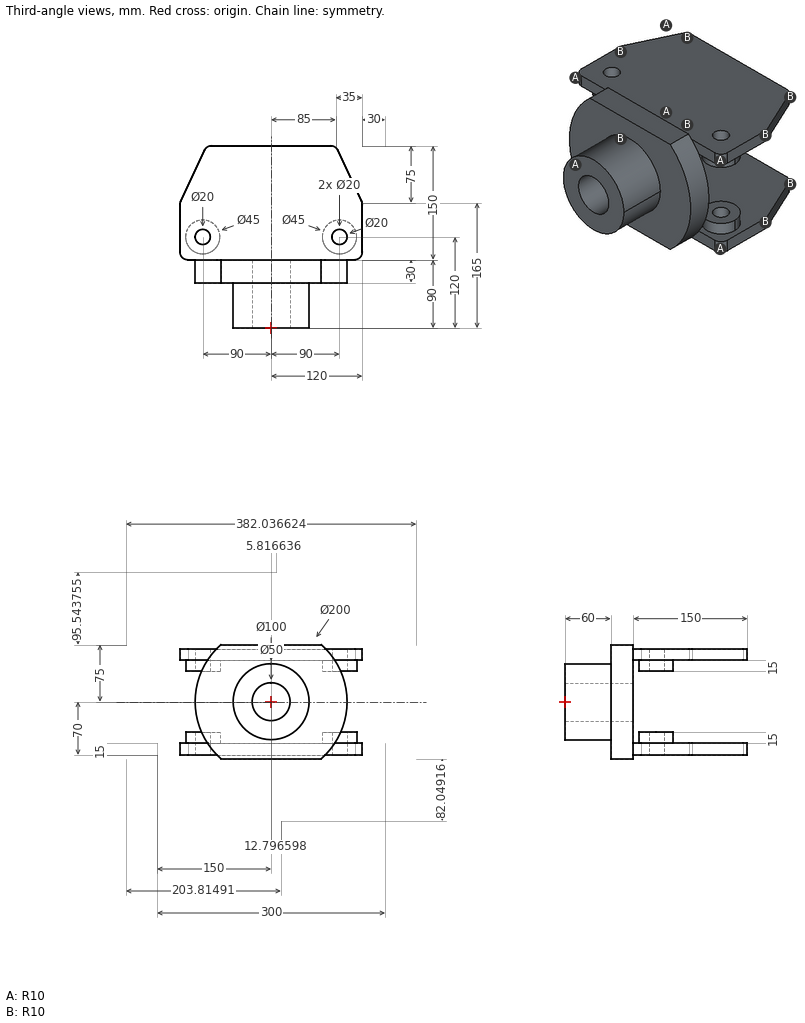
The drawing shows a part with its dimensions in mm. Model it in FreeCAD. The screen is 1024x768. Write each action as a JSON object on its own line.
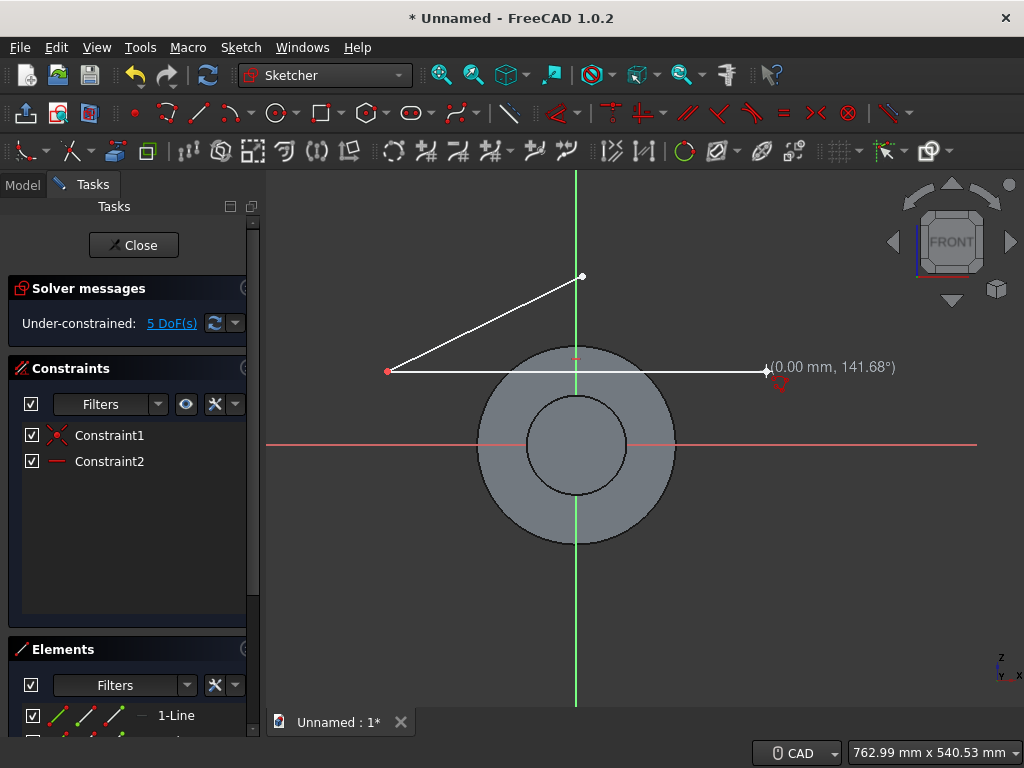
{"action": "scroll", "coordinate": [582, 276], "scroll_direction": "up", "scroll_amount": 6}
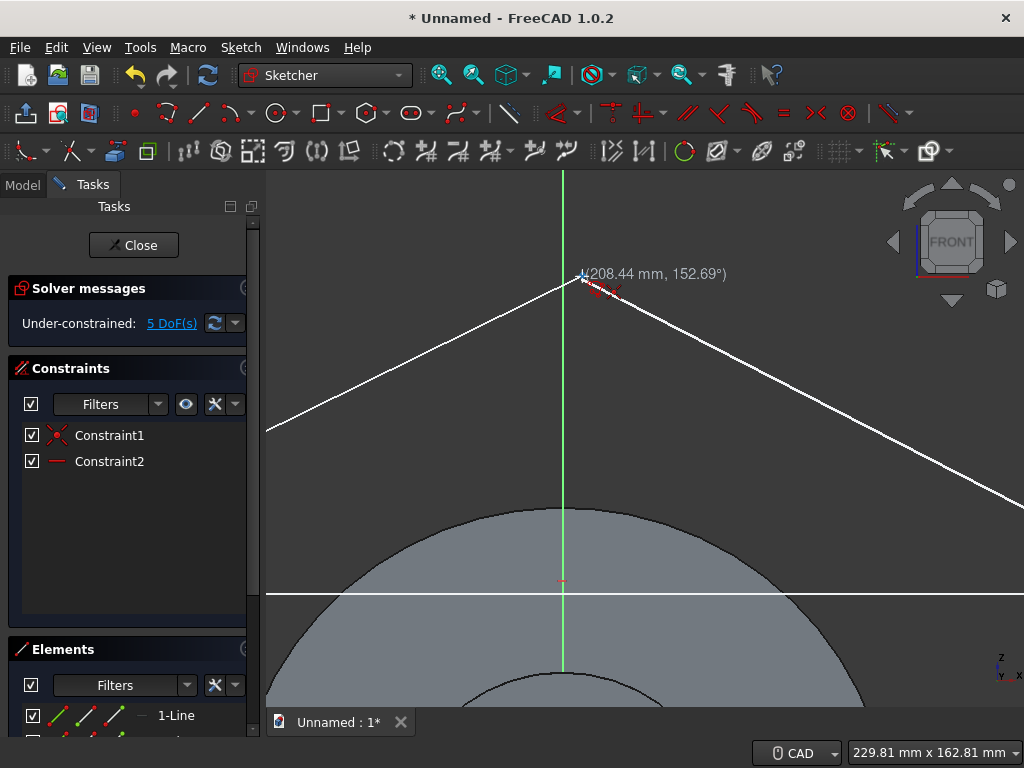
{"action": "left_click", "coordinate": [582, 276]}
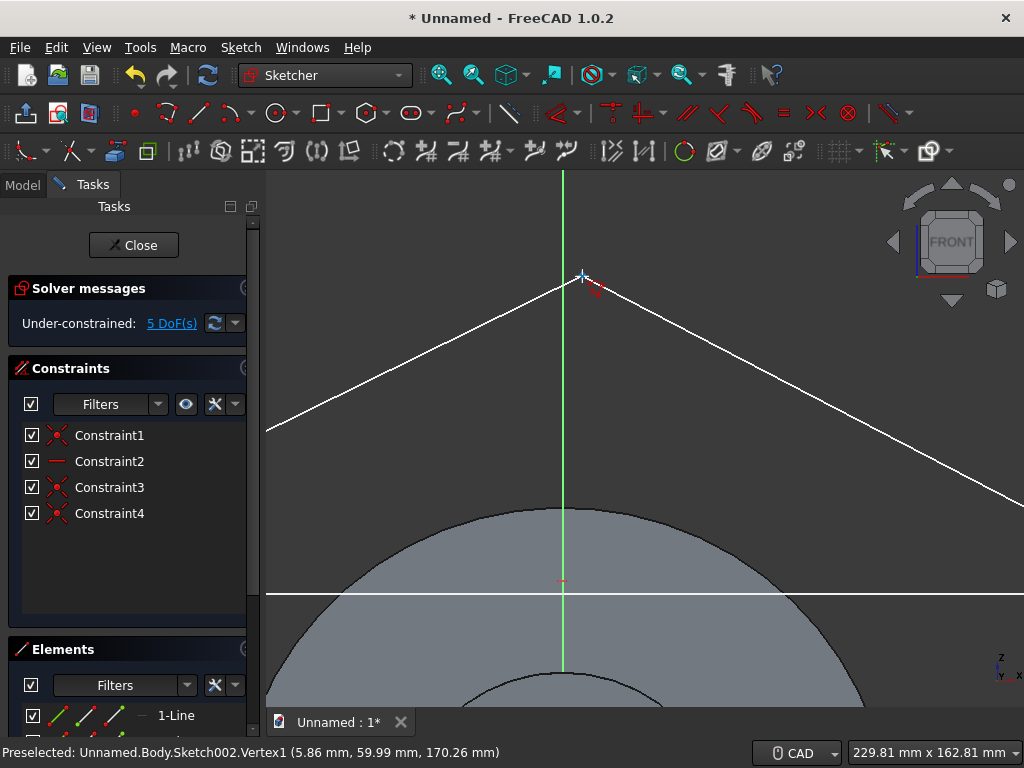
{"action": "scroll", "coordinate": [582, 276], "scroll_direction": "down", "scroll_amount": 6}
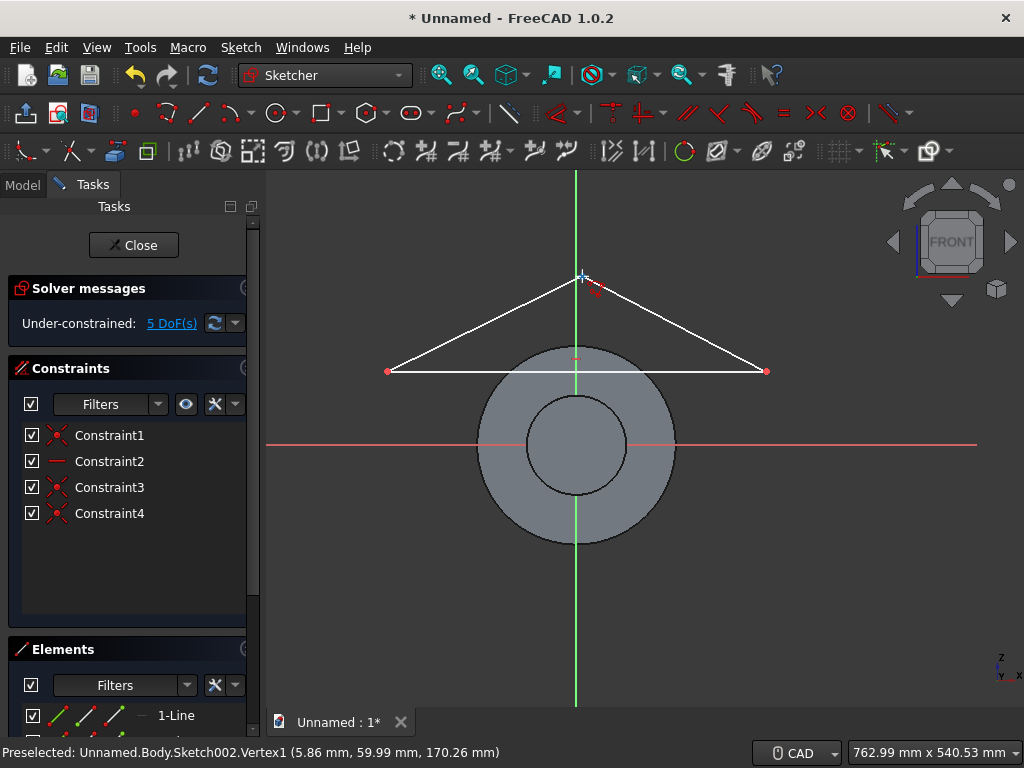
{"action": "scroll", "coordinate": [589, 601], "scroll_direction": "up", "scroll_amount": 2}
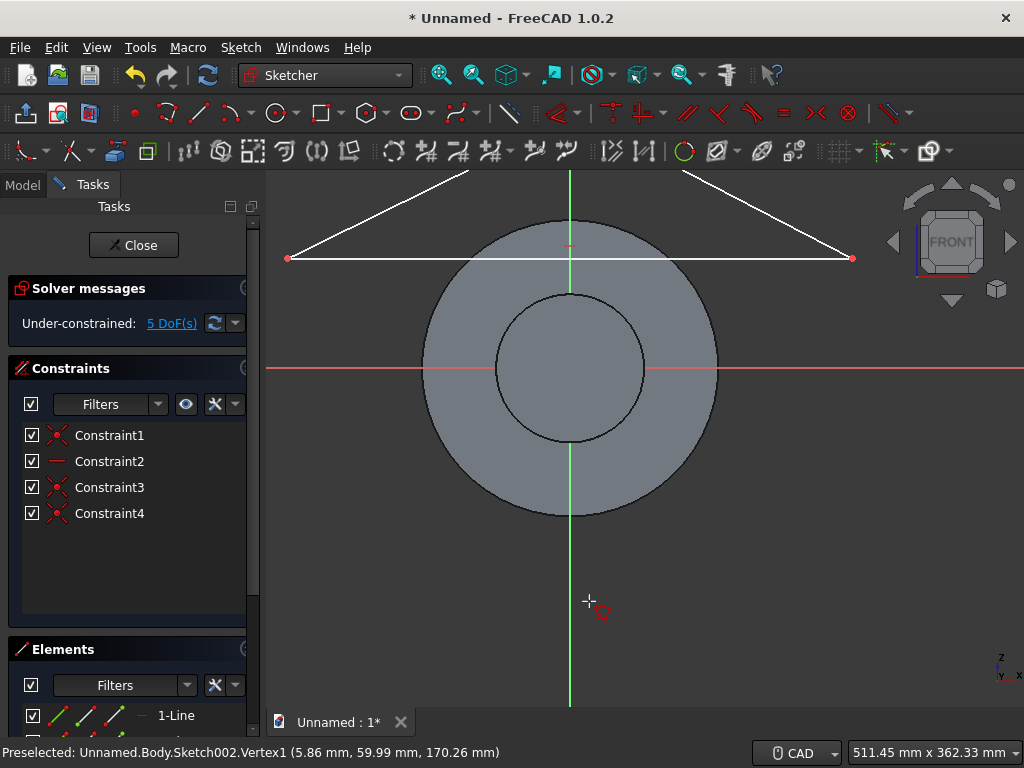
{"action": "left_click", "coordinate": [589, 601]}
{"action": "left_click", "coordinate": [853, 479]}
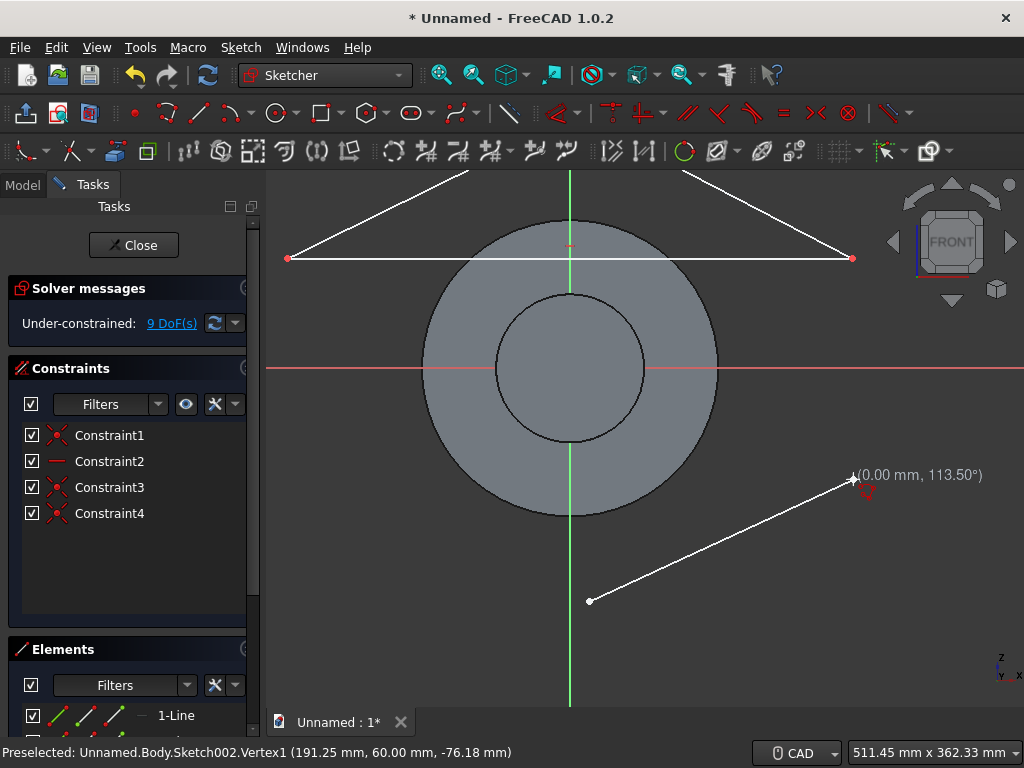
{"action": "scroll", "coordinate": [590, 602], "scroll_direction": "down", "scroll_amount": 2}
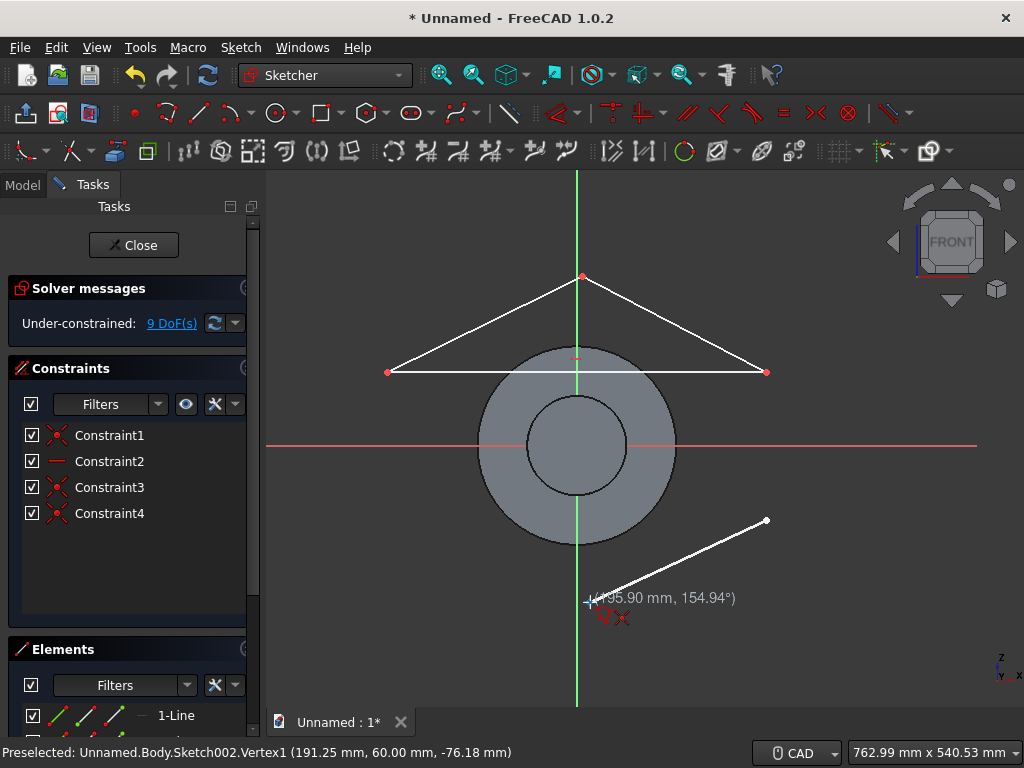
{"action": "left_click", "coordinate": [387, 520]}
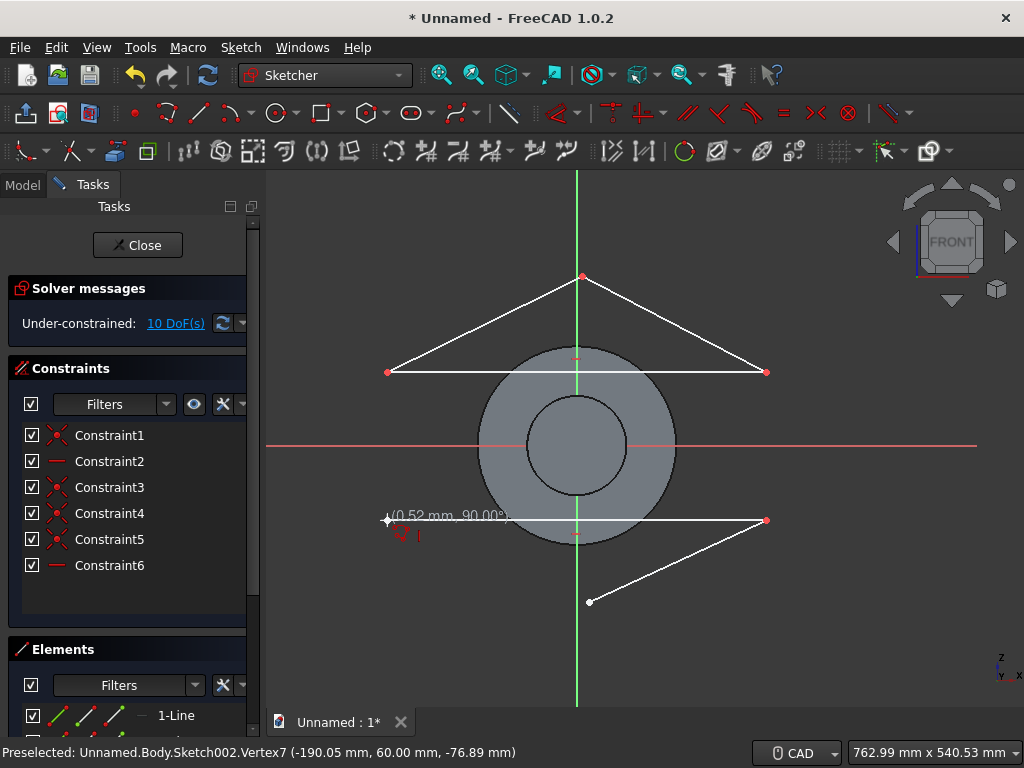
{"action": "scroll", "coordinate": [590, 602], "scroll_direction": "up", "scroll_amount": 2}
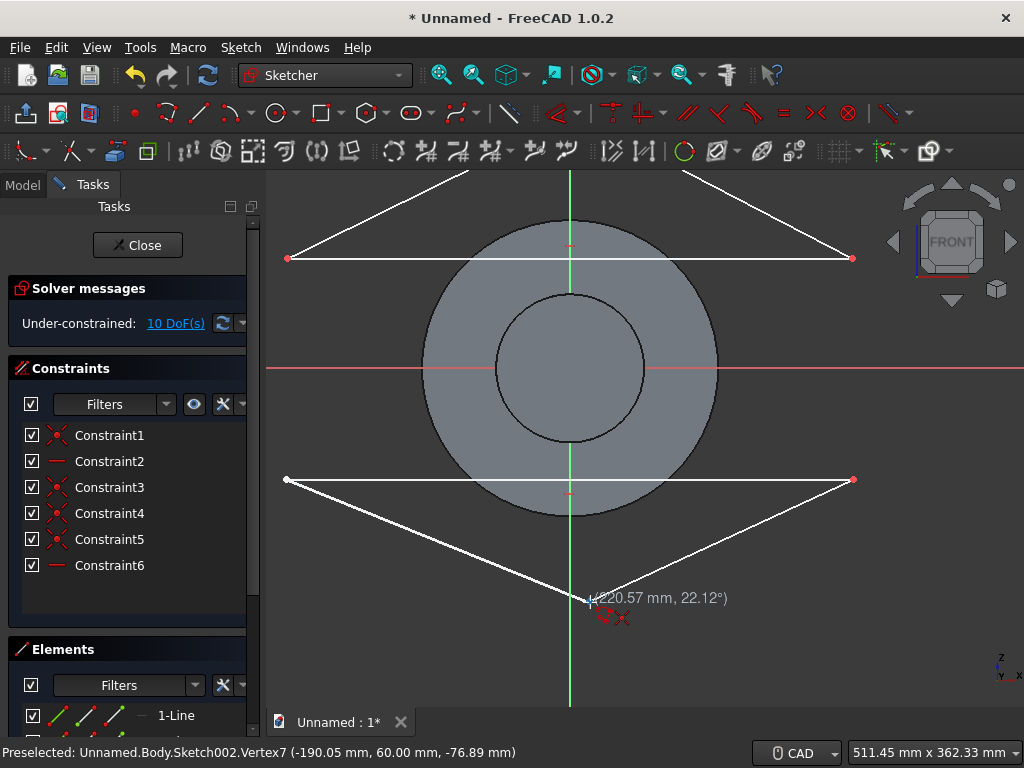
{"action": "left_click", "coordinate": [589, 602]}
{"action": "key", "text": "Escape"}
{"action": "key", "text": "Escape"}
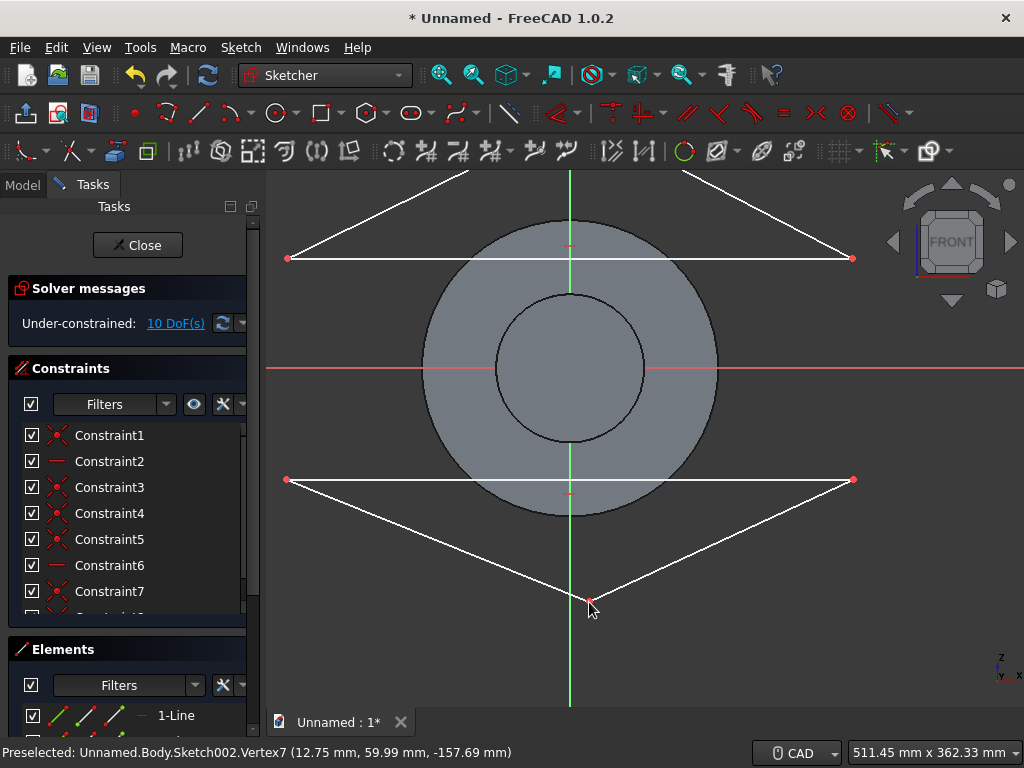
{"action": "left_click", "coordinate": [853, 259]}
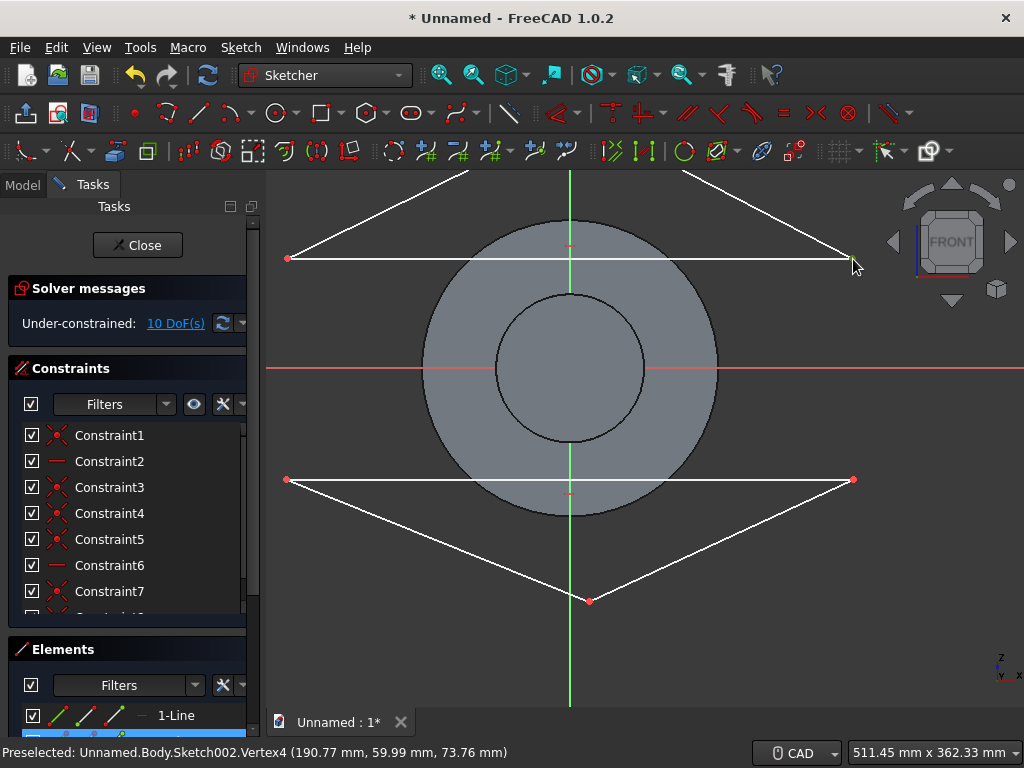
{"action": "left_click", "coordinate": [853, 480]}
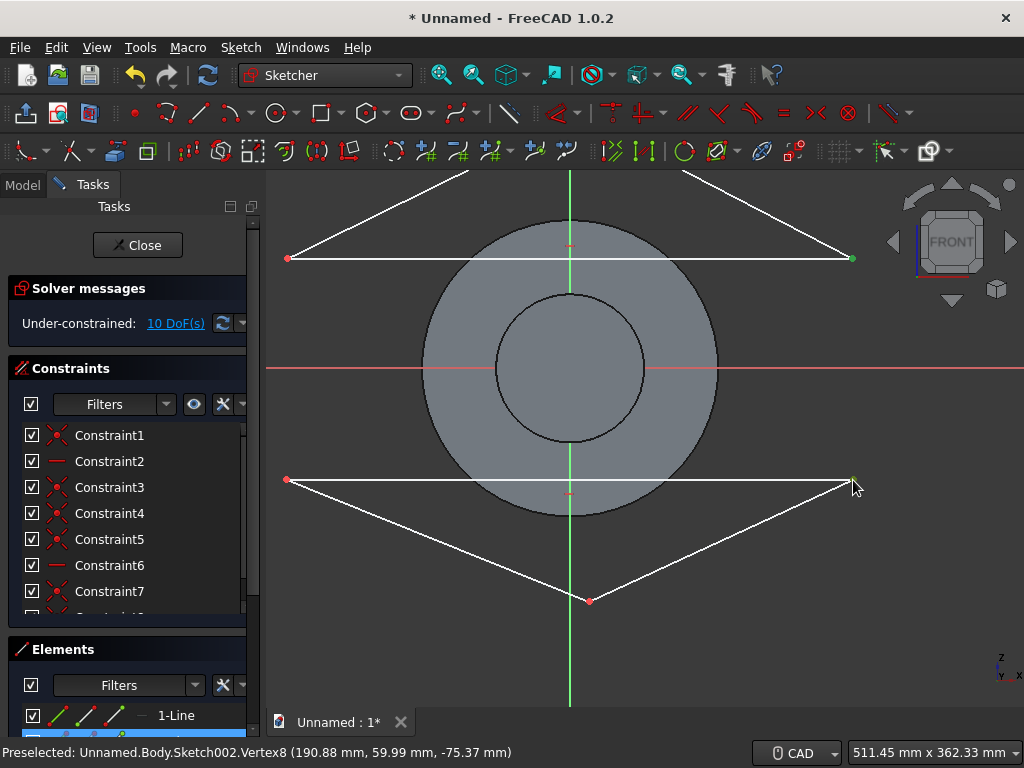
{"action": "left_click", "coordinate": [334, 368]}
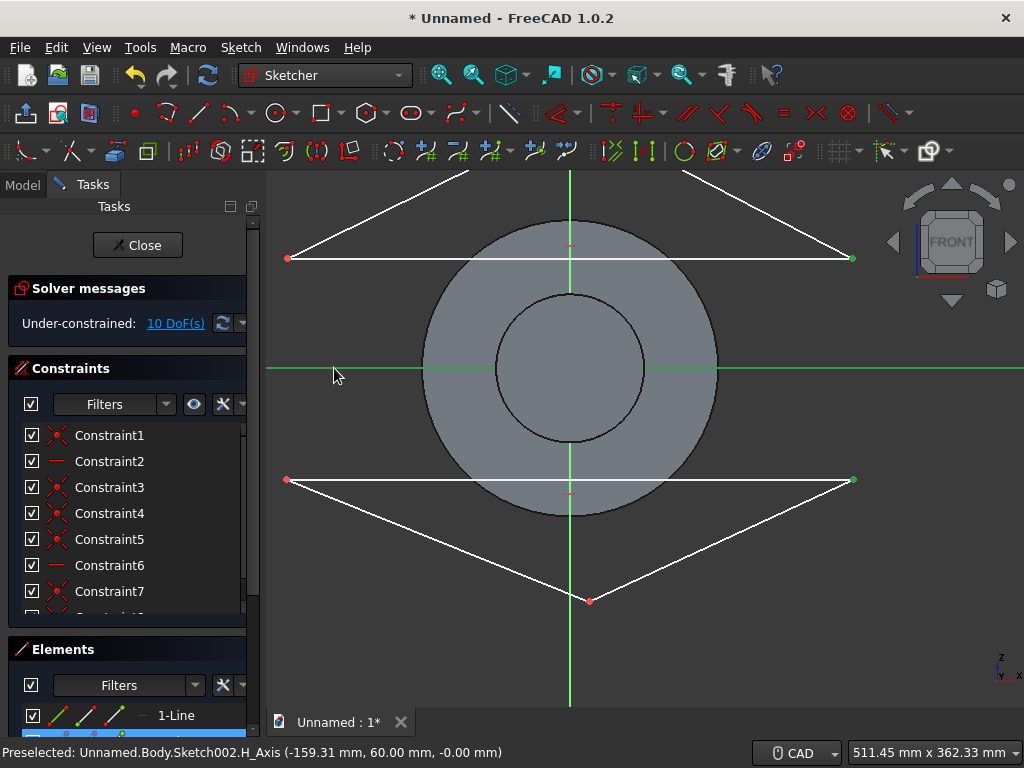
{"action": "left_click", "coordinate": [816, 114]}